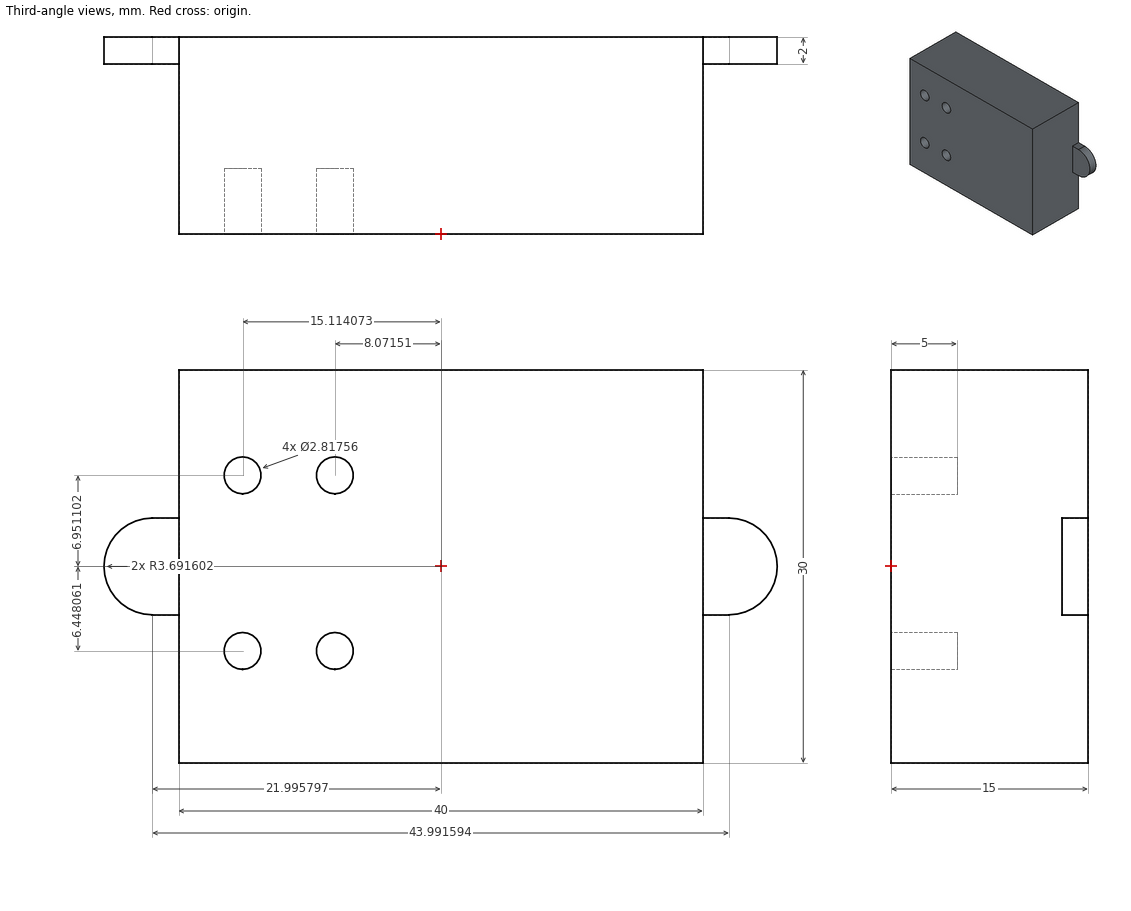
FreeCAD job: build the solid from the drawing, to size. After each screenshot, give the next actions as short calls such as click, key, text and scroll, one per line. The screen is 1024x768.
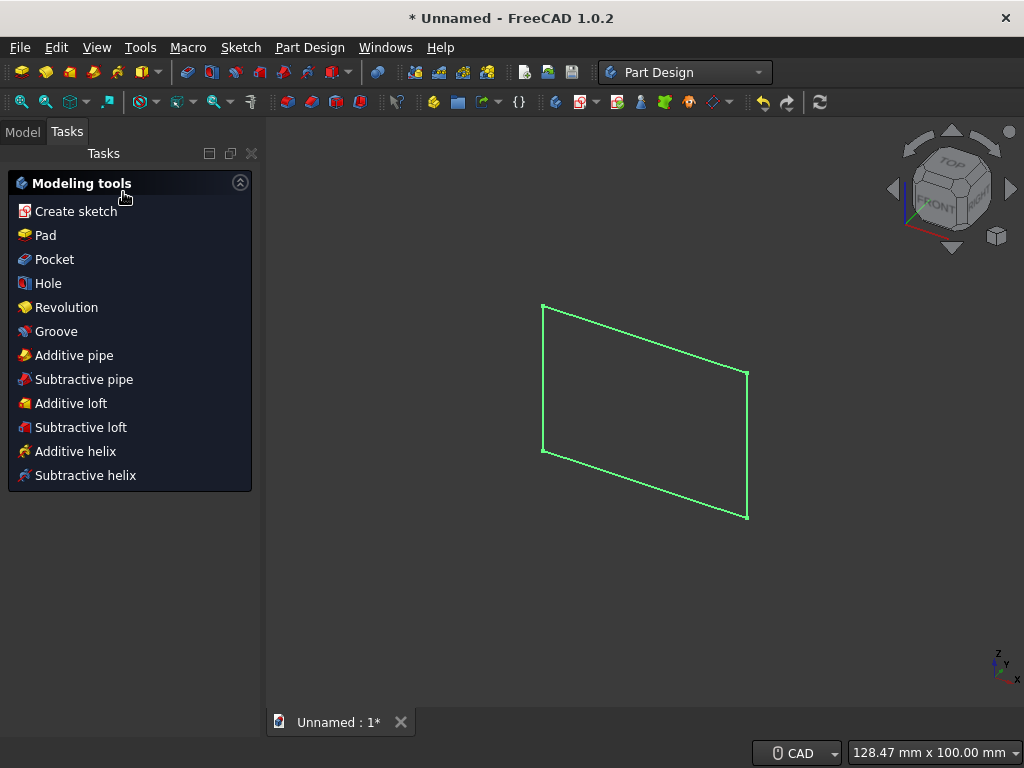
click(22, 72)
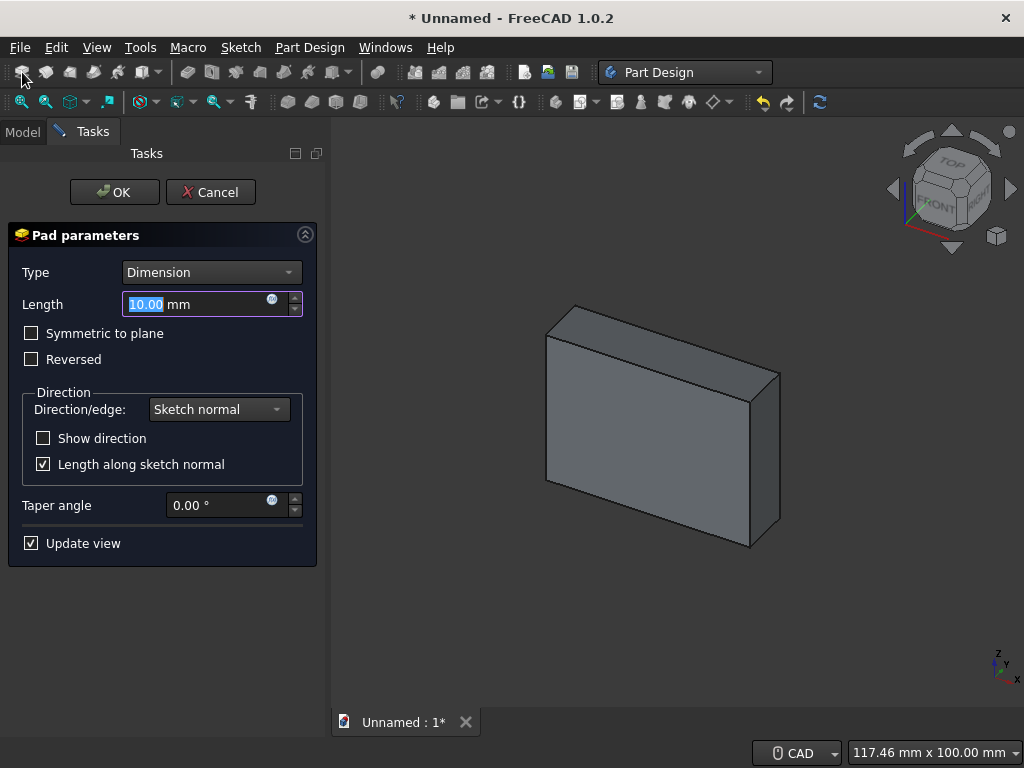
text(15)
key(Tab)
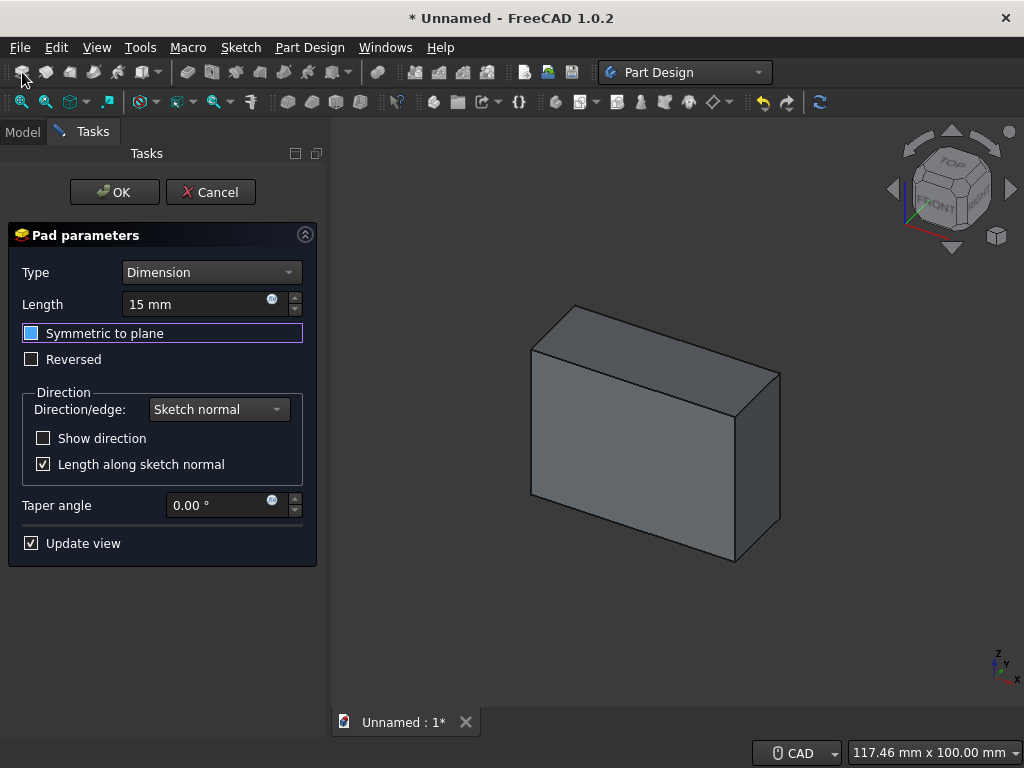
click(30, 359)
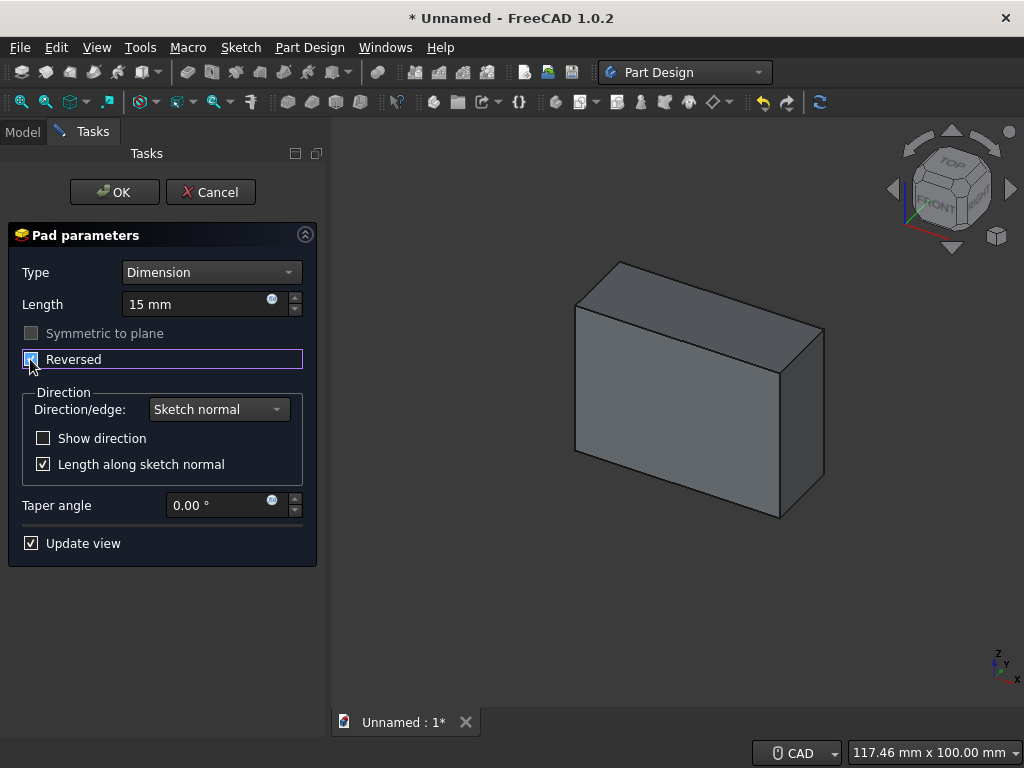
click(115, 192)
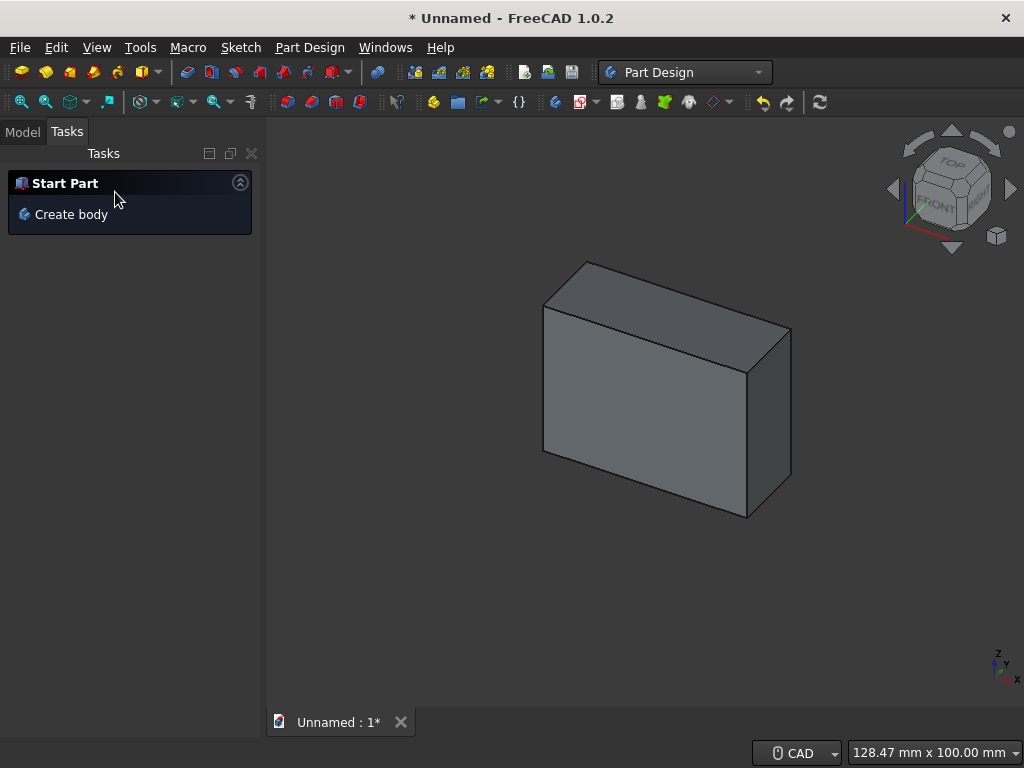
key(v)
key(f)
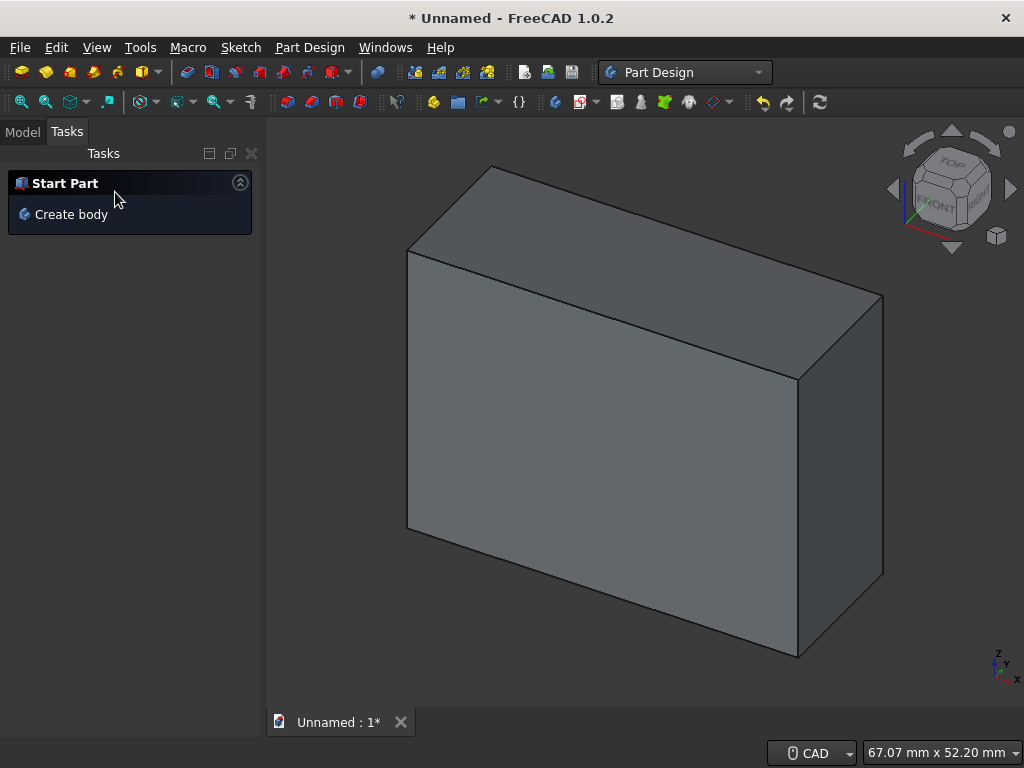
key(4)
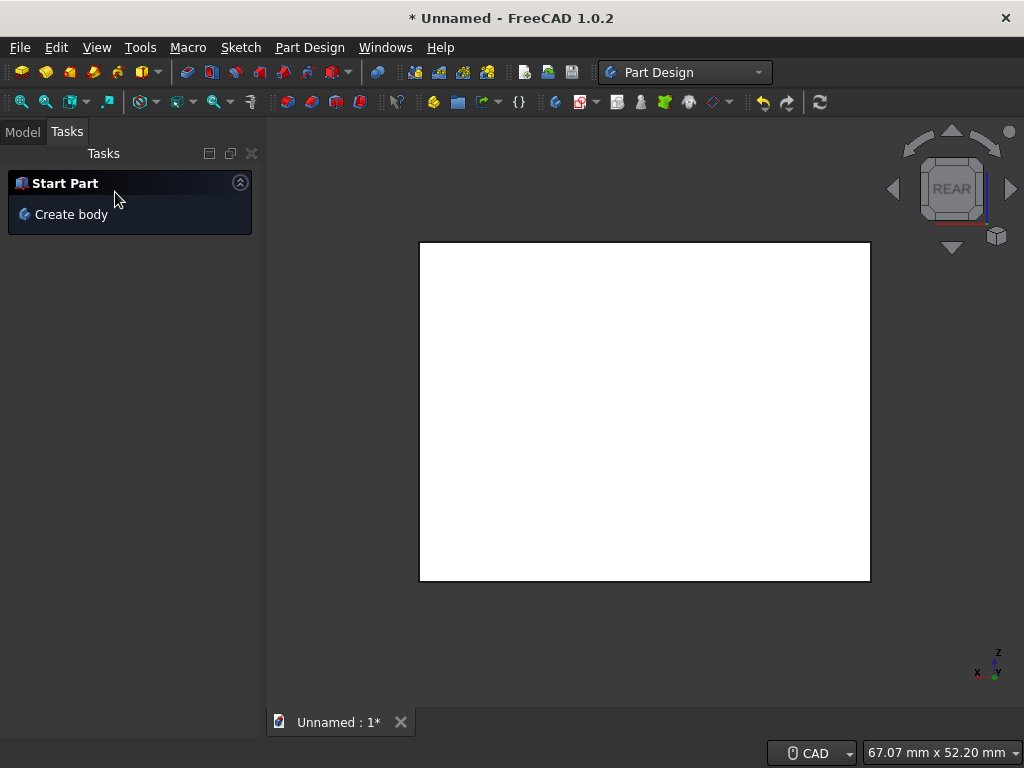
click(645, 411)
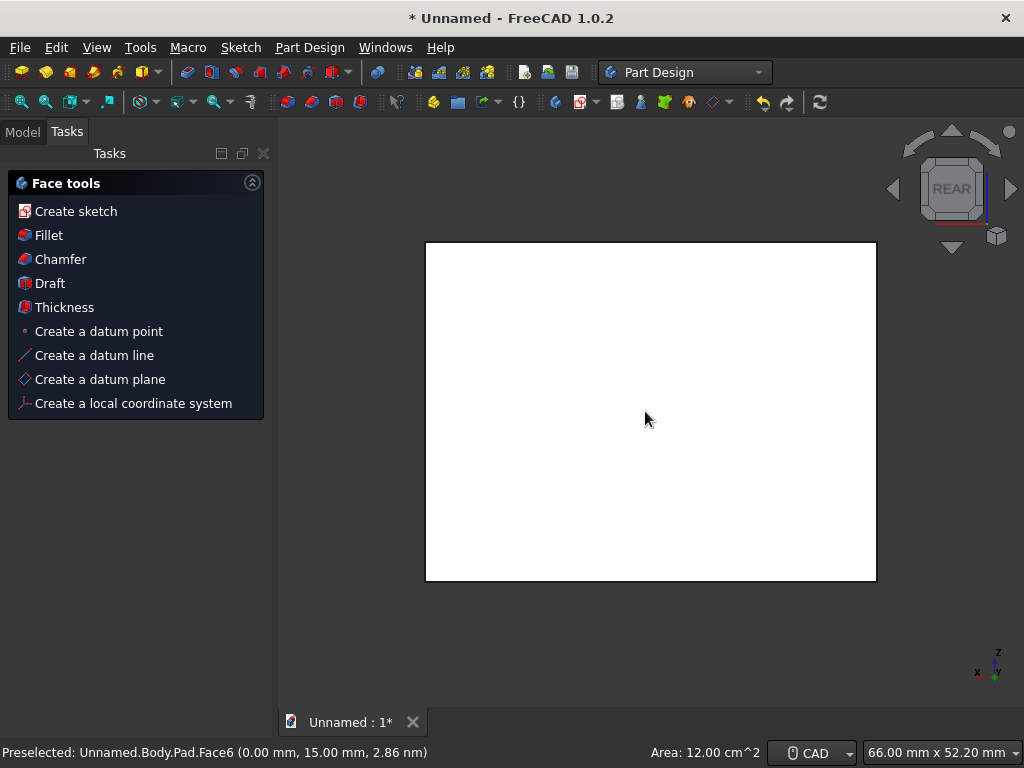
click(580, 102)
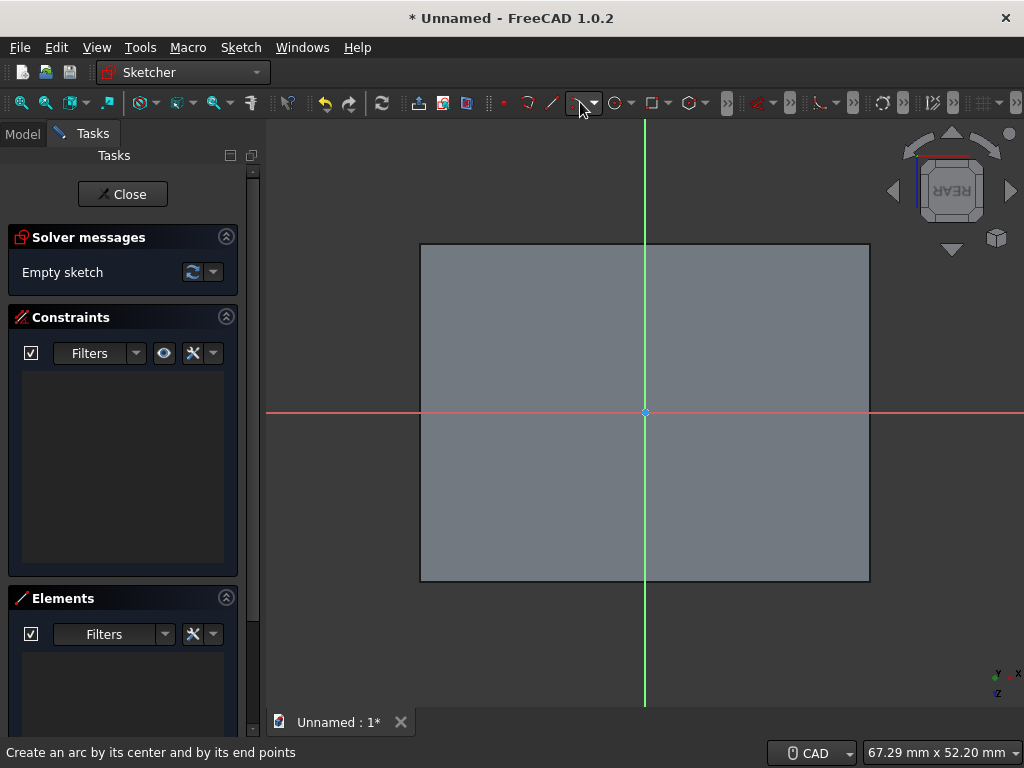
scroll(437, 413, down, 2)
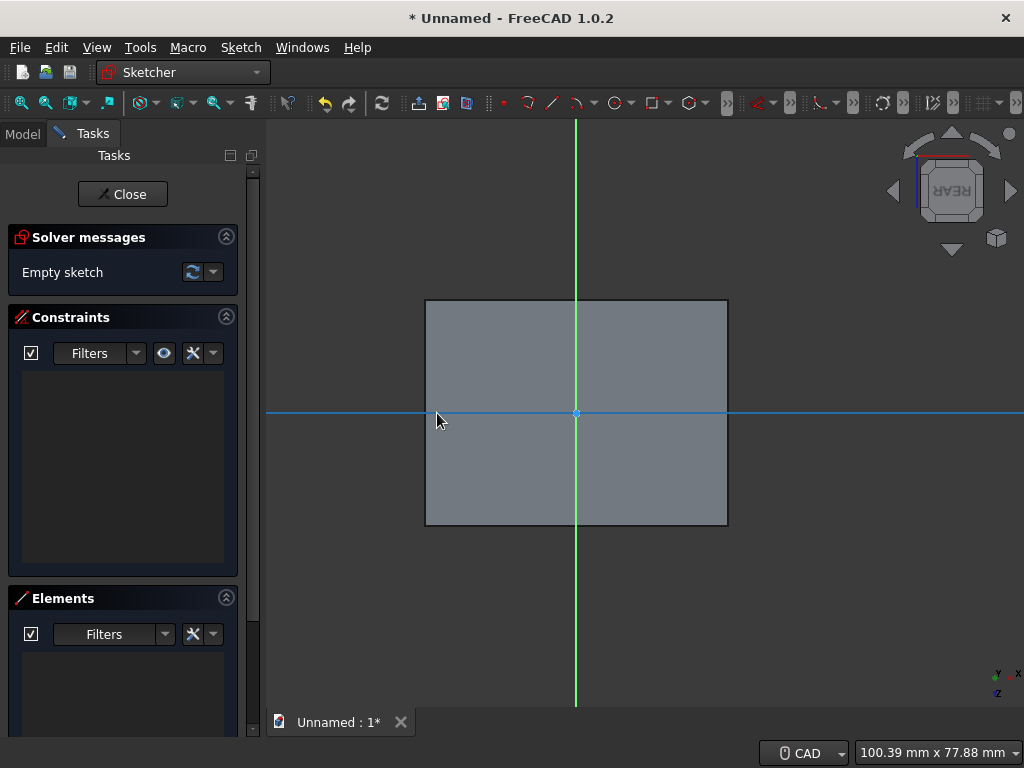
key(g)
key(s)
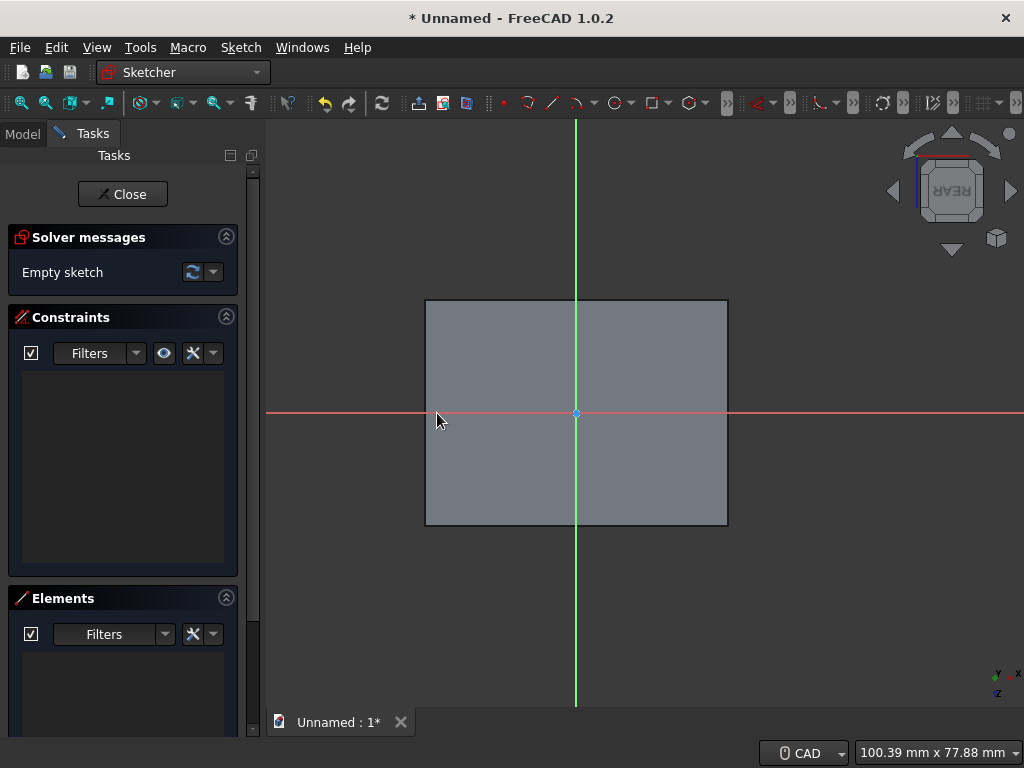
click(410, 413)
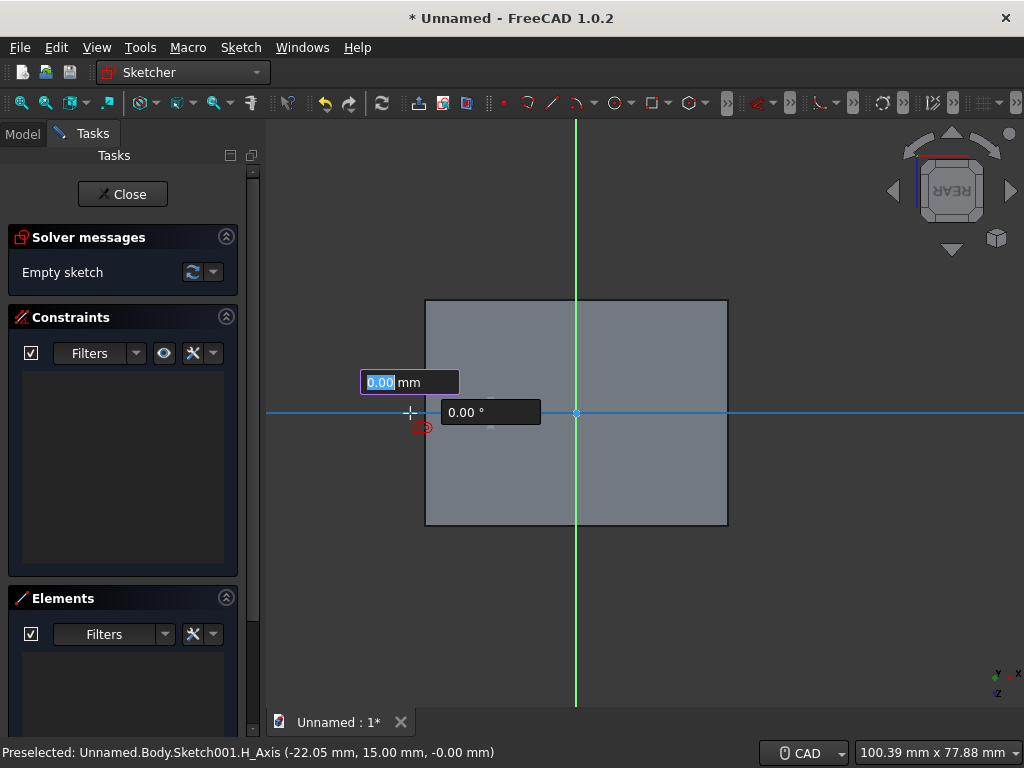
click(743, 404)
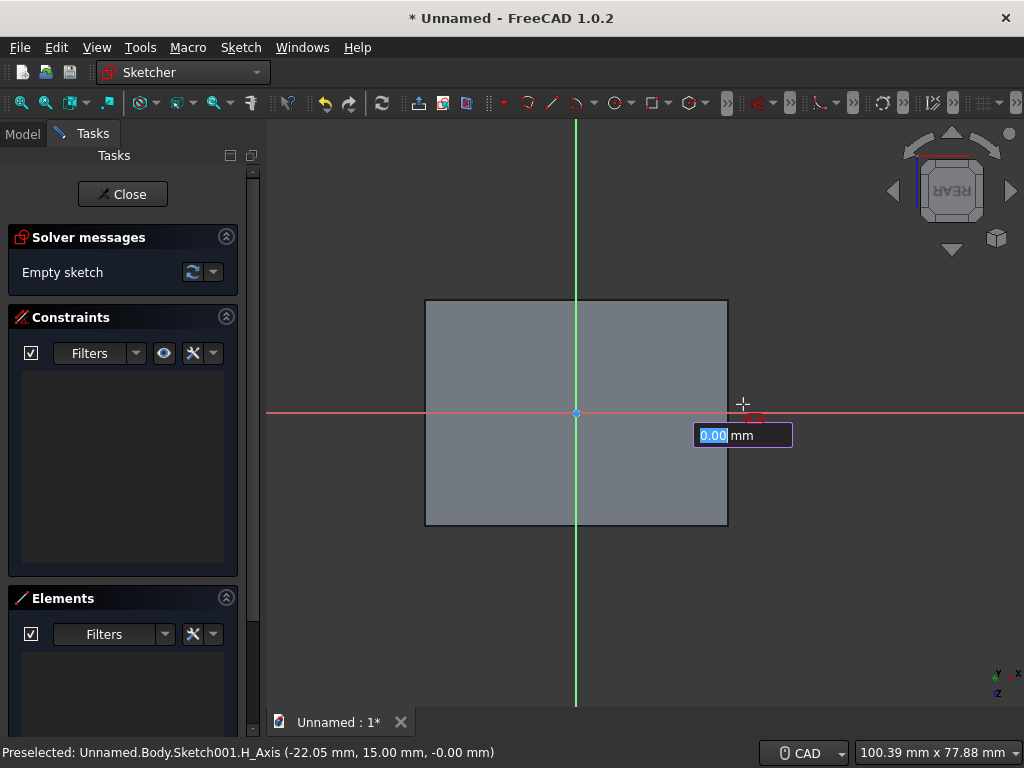
click(626, 385)
key(Escape)